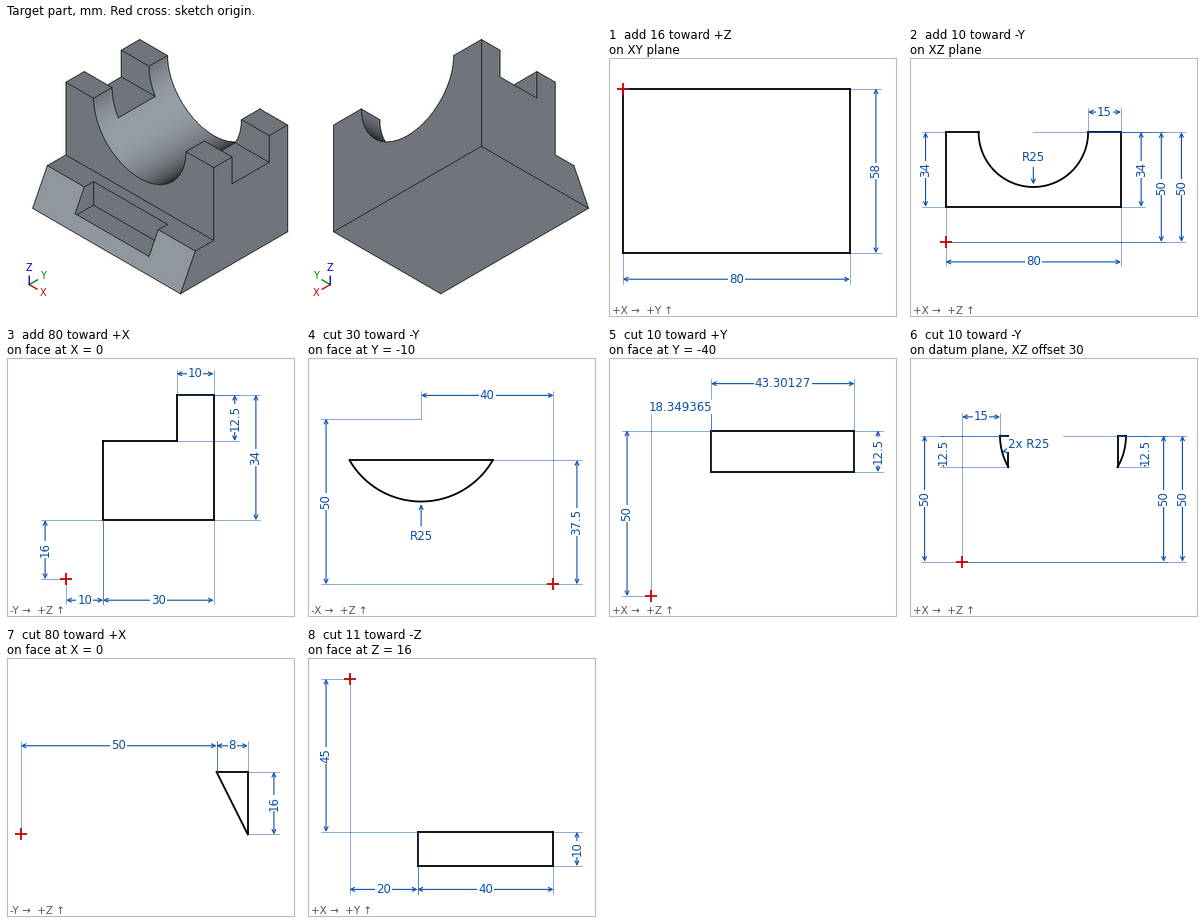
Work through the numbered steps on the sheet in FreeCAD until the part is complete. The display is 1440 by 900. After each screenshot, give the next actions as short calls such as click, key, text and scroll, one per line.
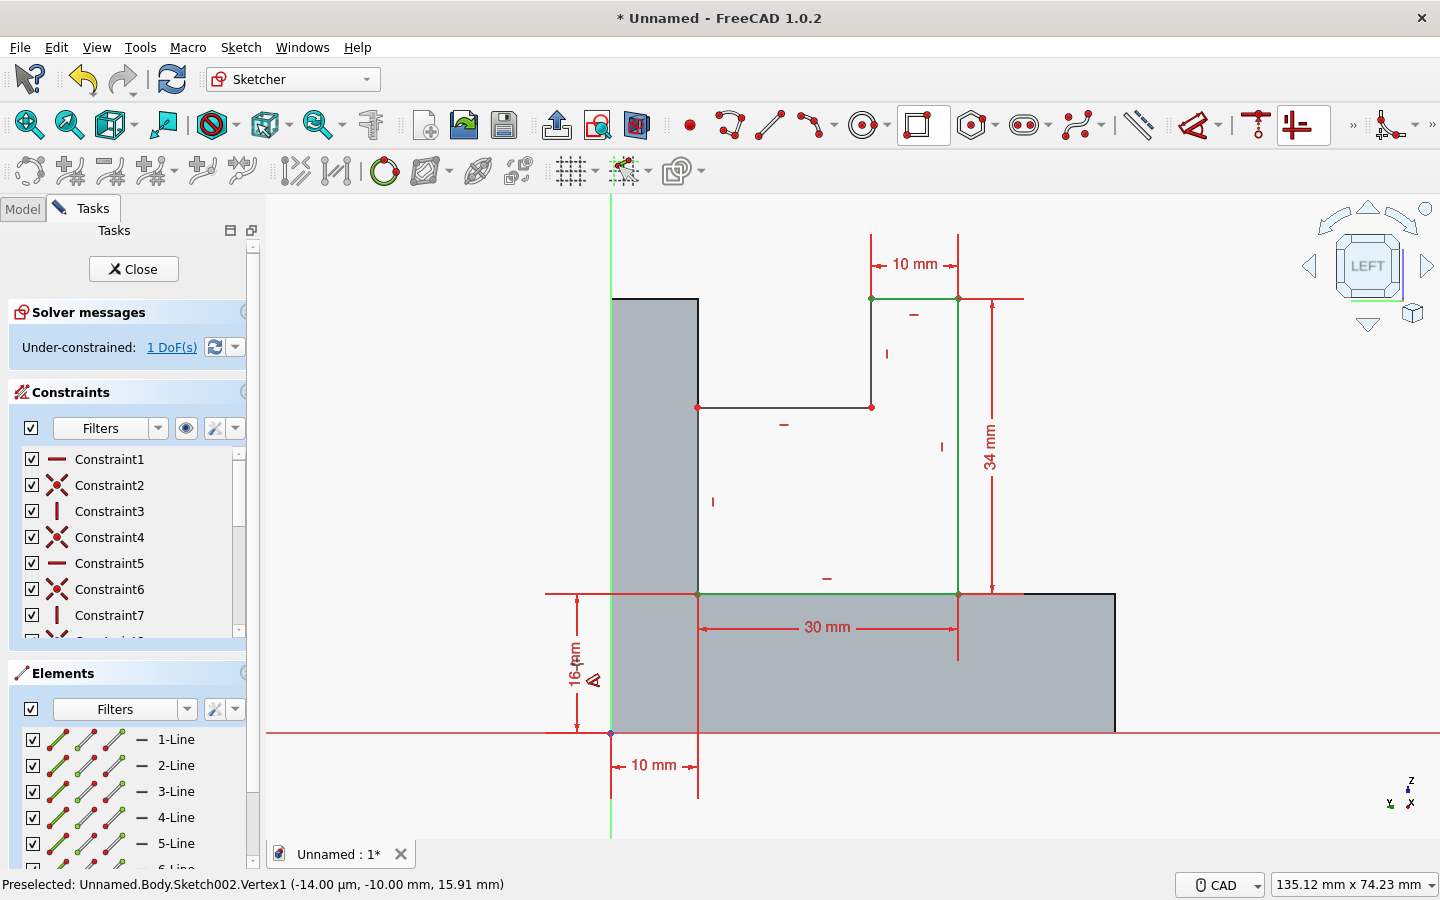
click(871, 332)
click(905, 353)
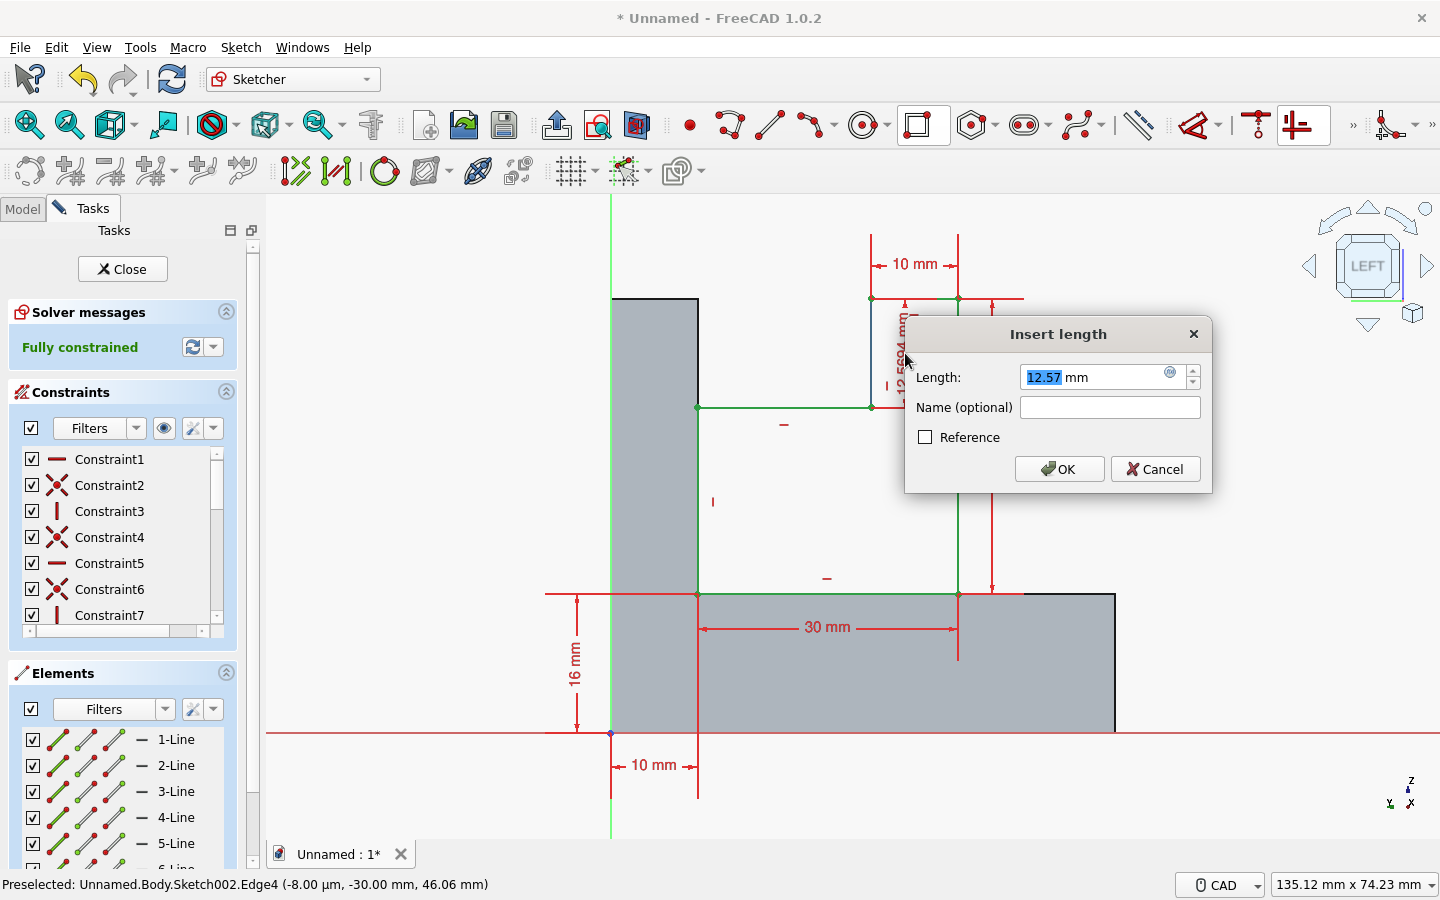
text(12.5)
key(Return)
key(Escape)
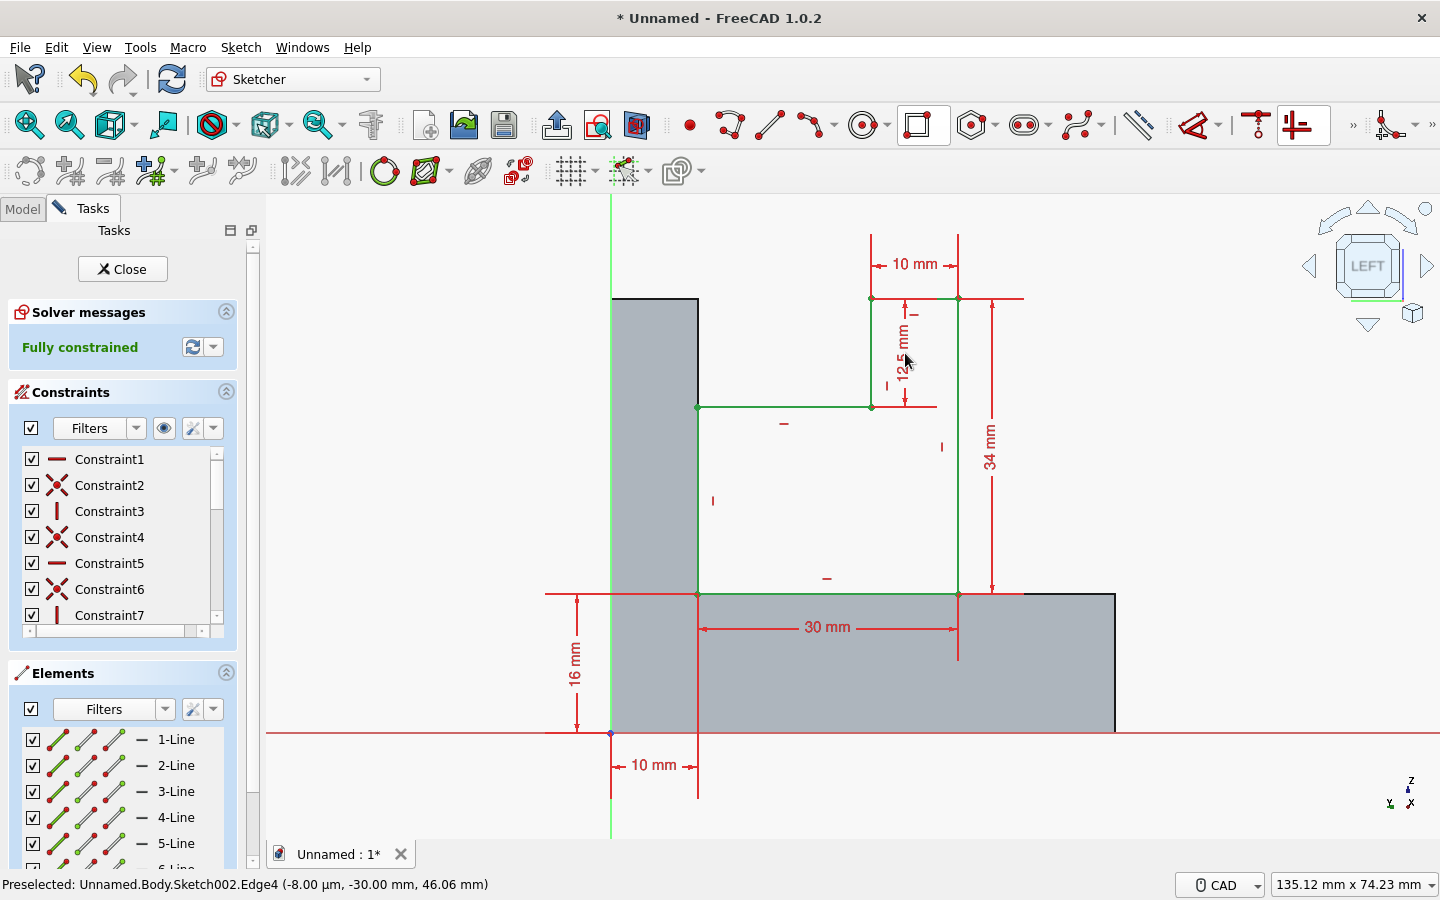
click(123, 269)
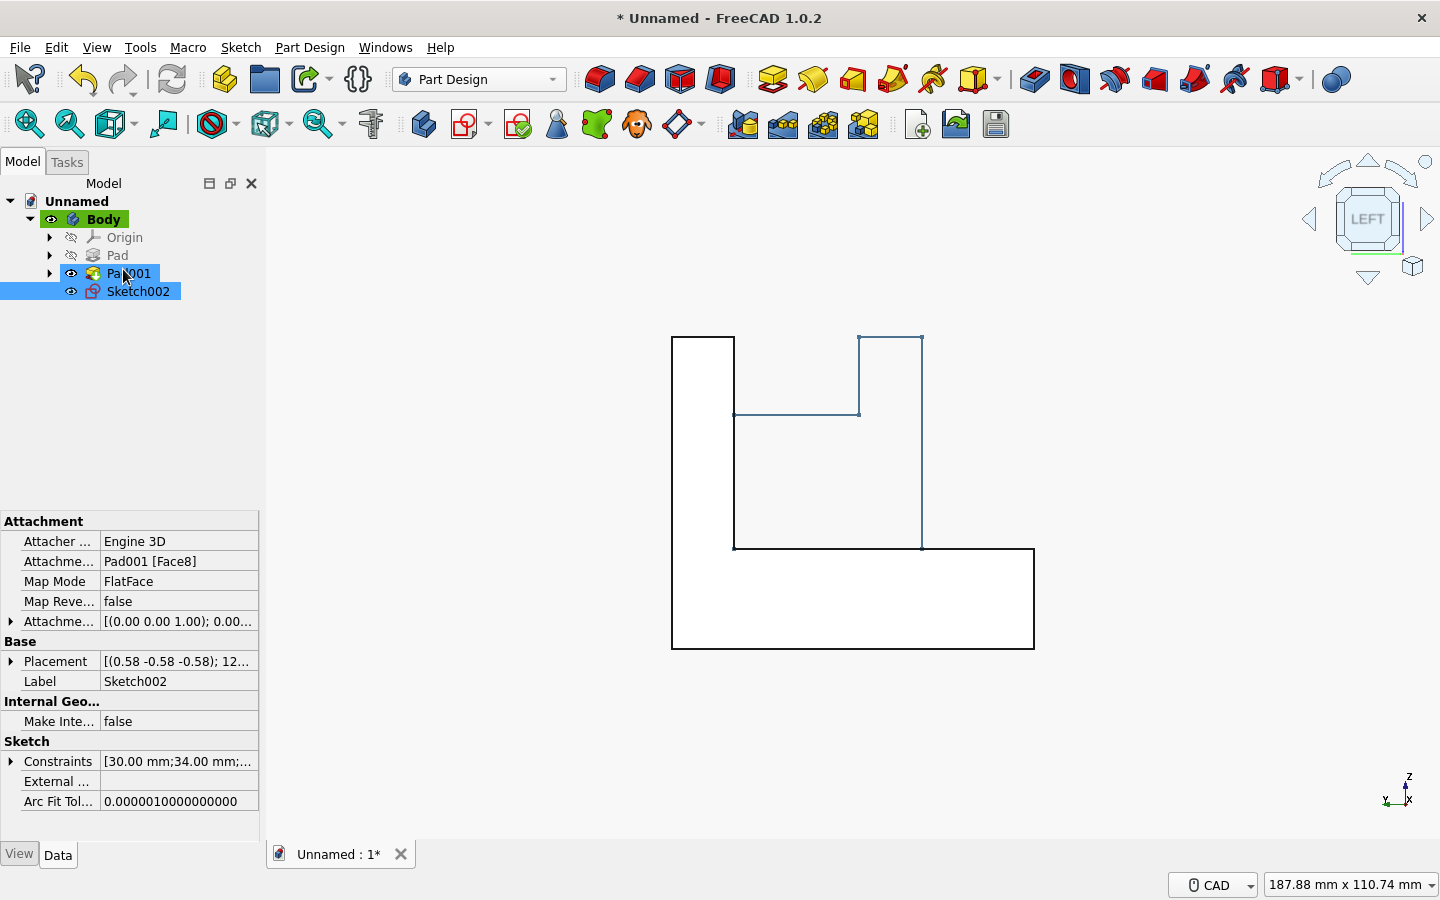
click(774, 80)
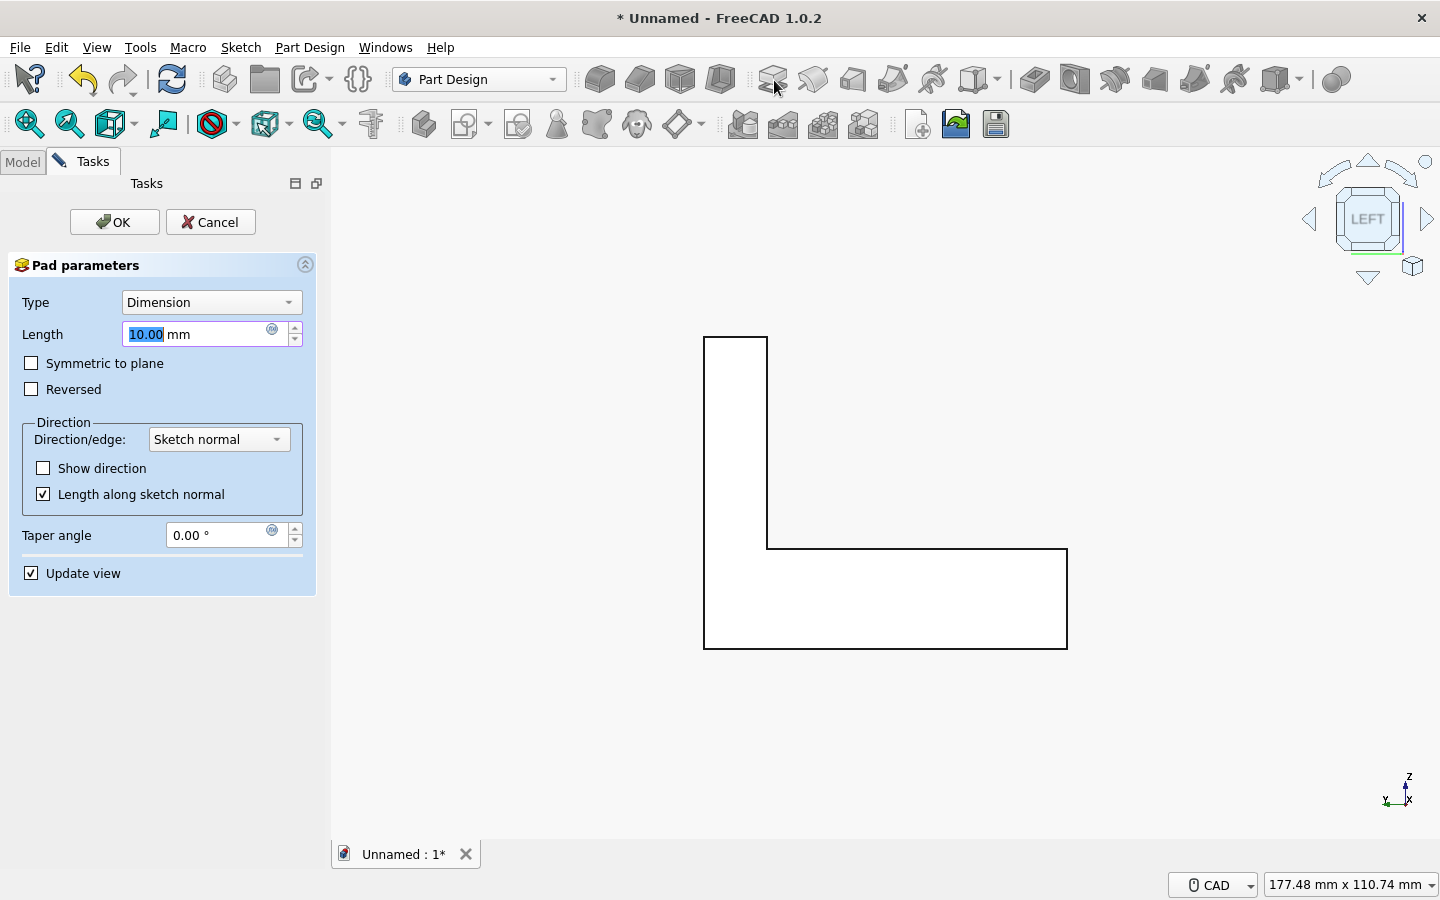
text(80)
key(Tab)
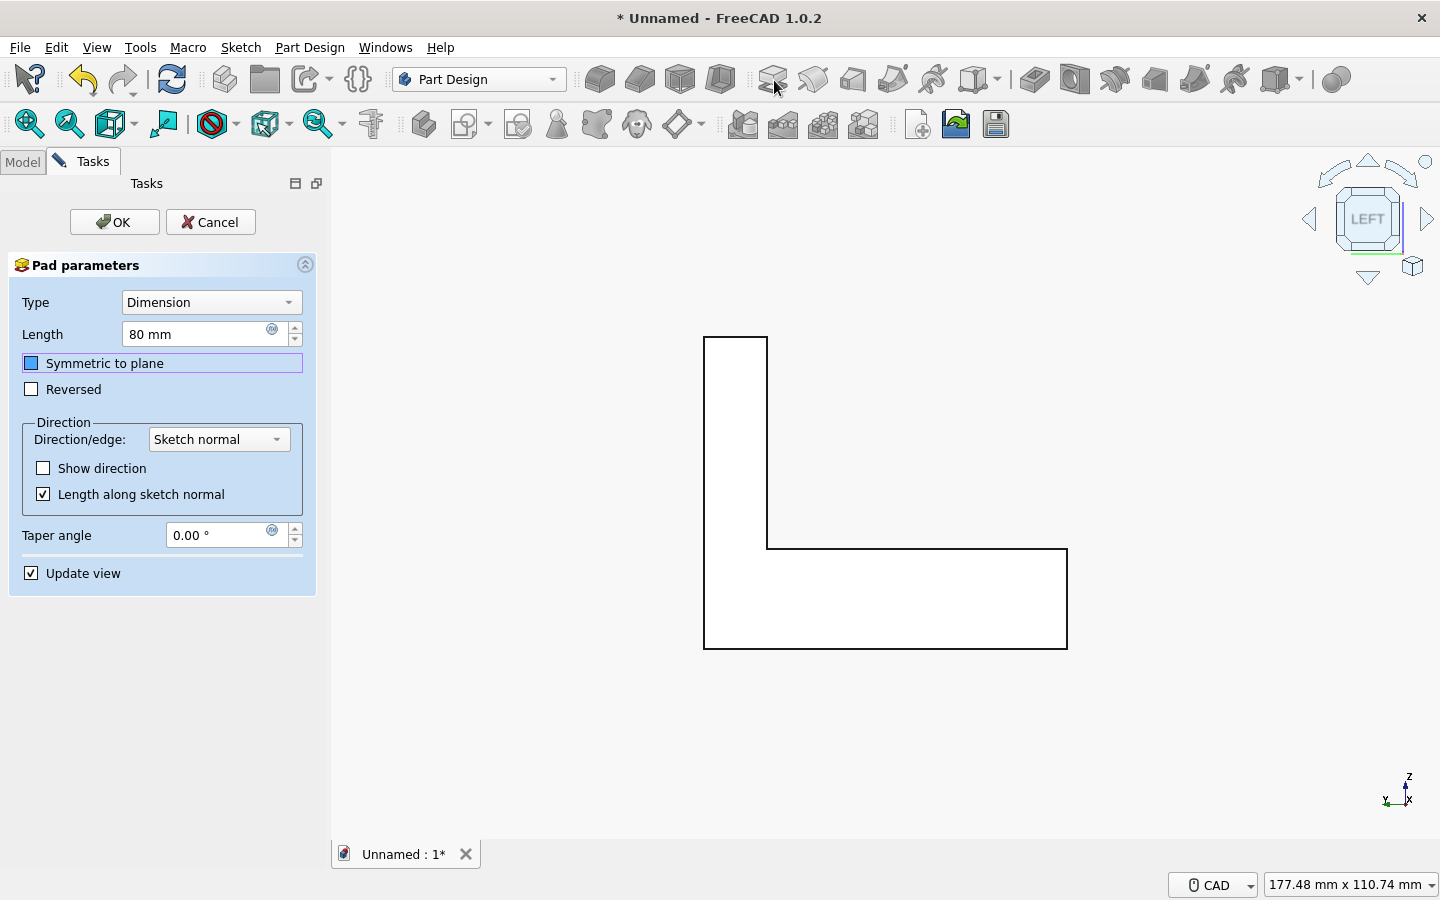
click(30, 389)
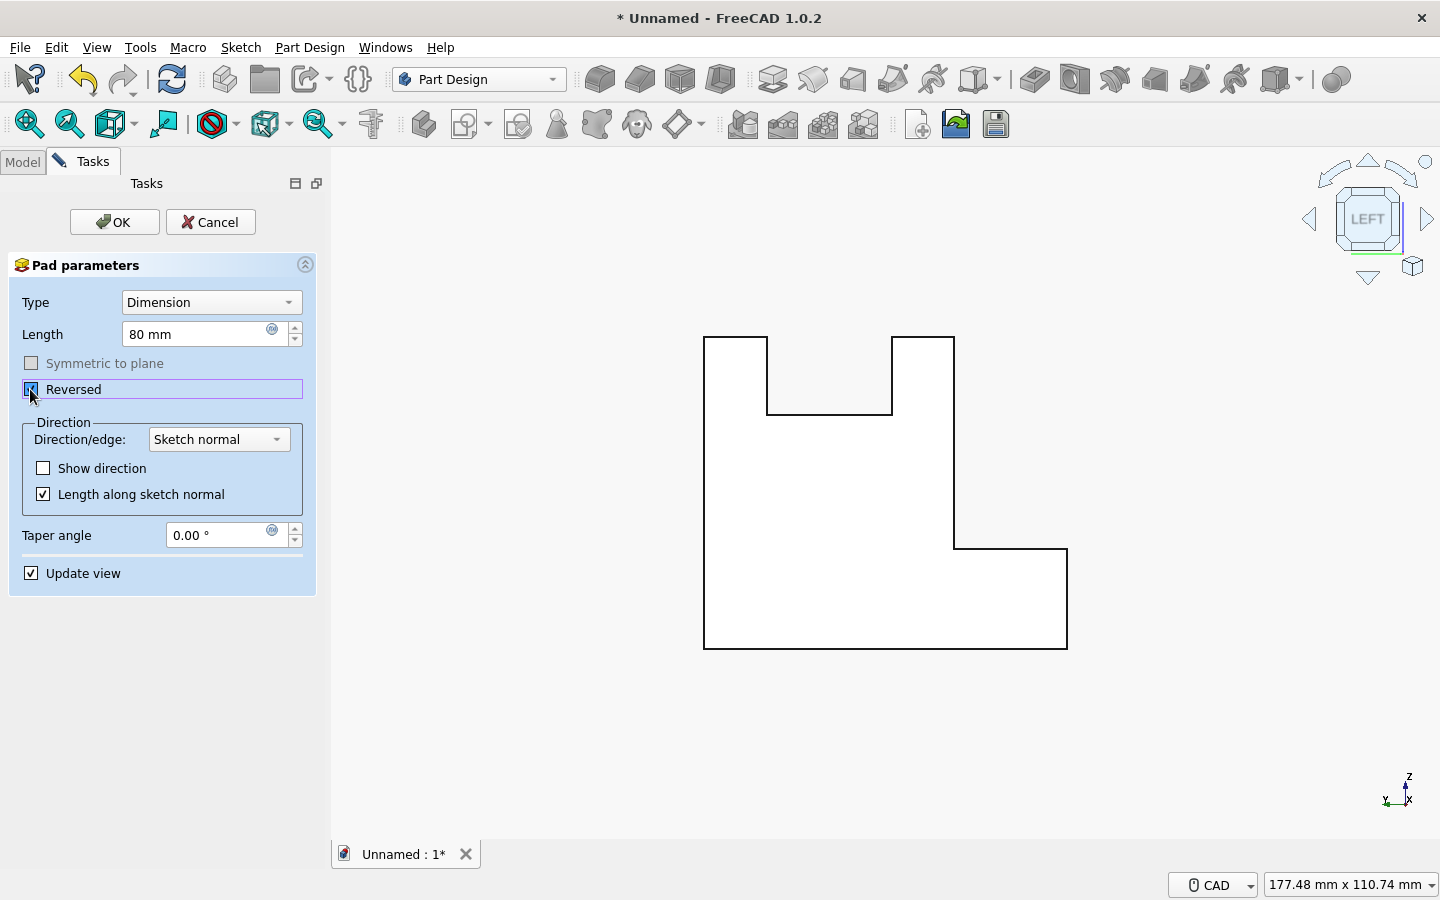
click(115, 222)